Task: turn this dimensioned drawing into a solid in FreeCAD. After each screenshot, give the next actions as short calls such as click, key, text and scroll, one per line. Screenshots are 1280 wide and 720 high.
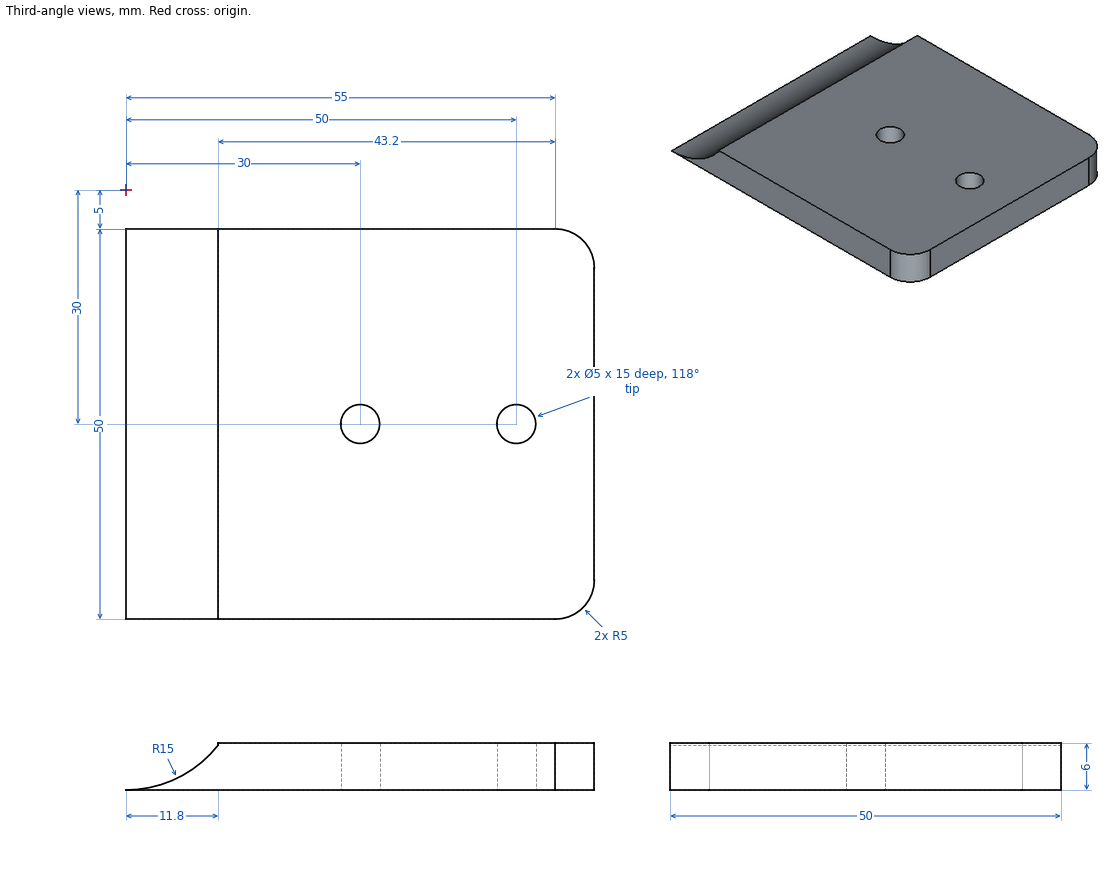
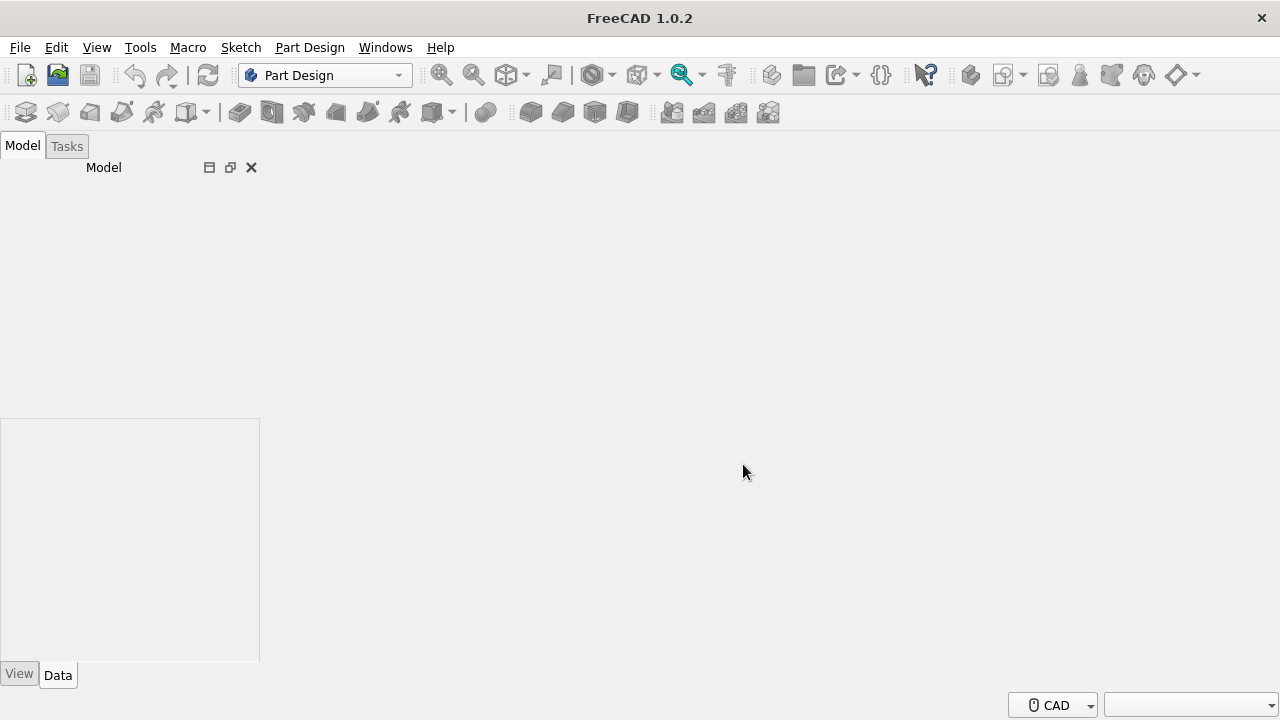
click(26, 76)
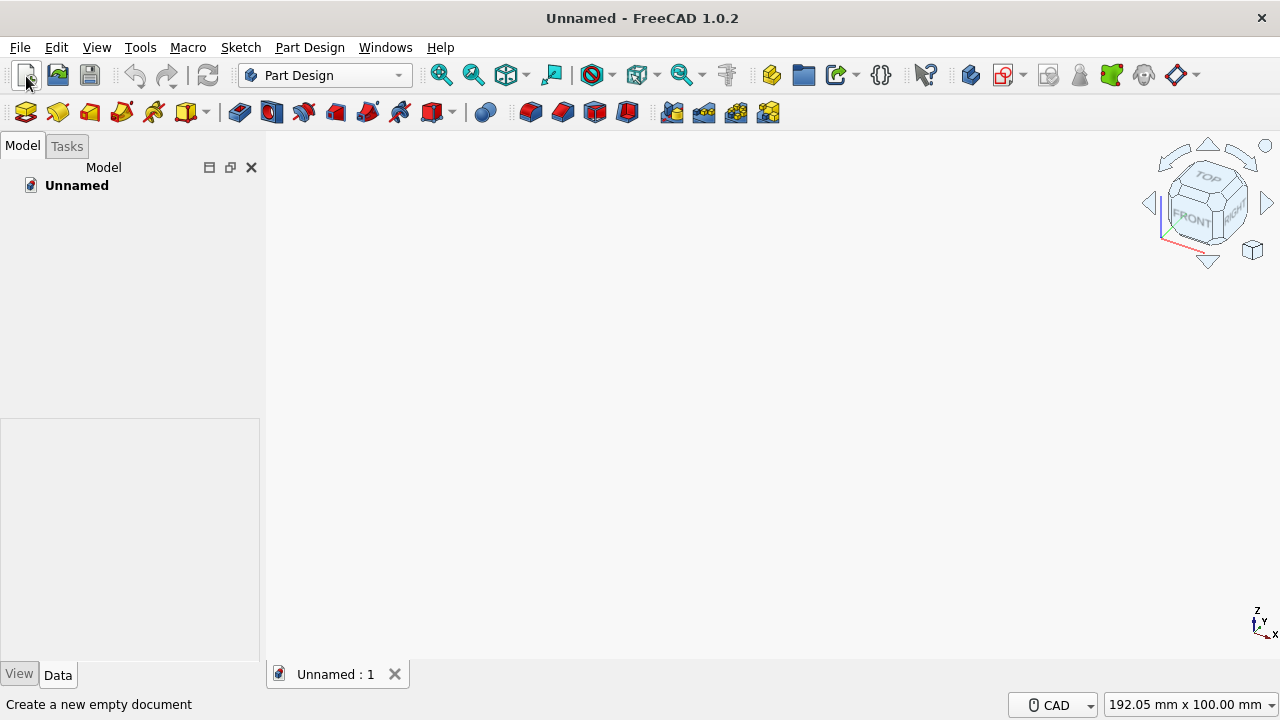
click(972, 76)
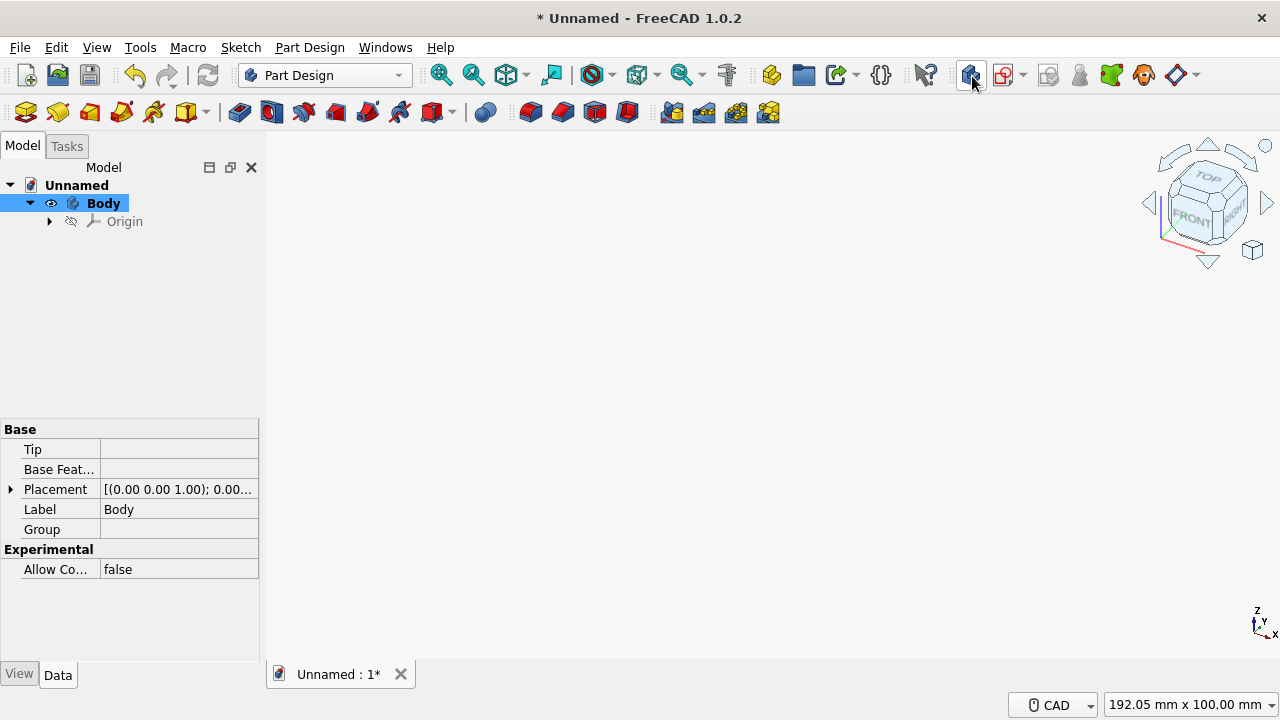
click(50, 221)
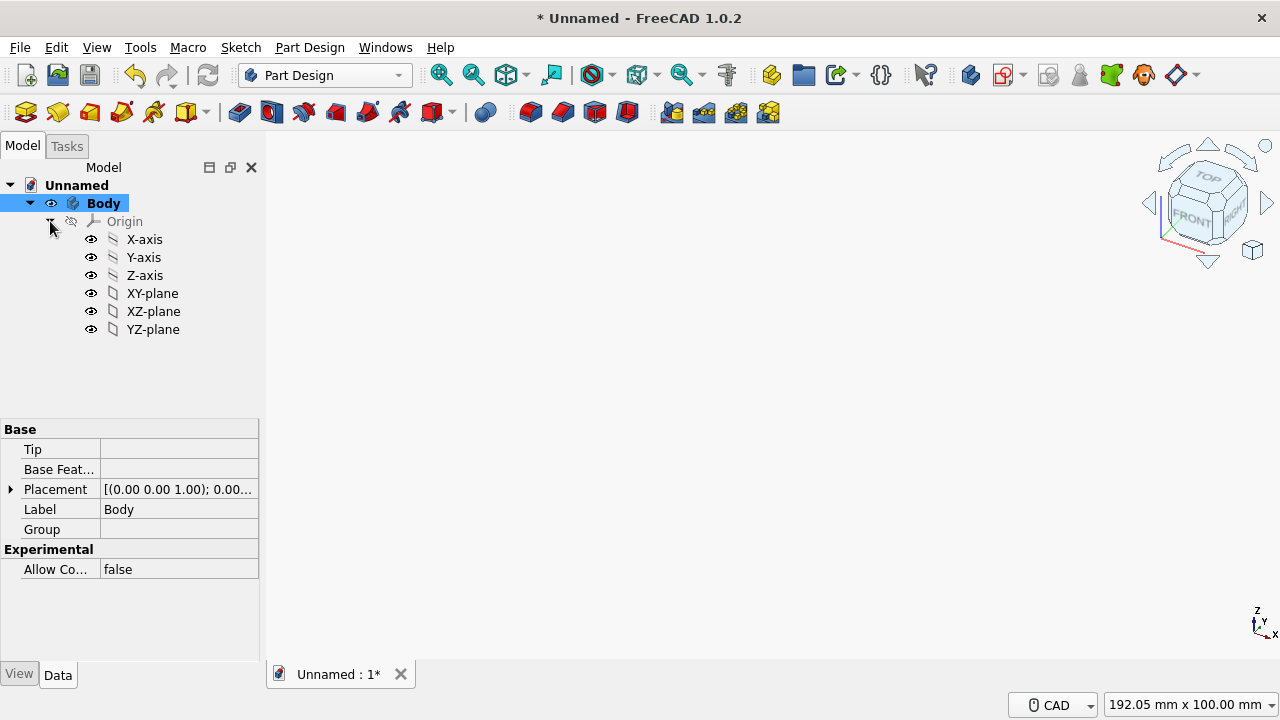
click(136, 293)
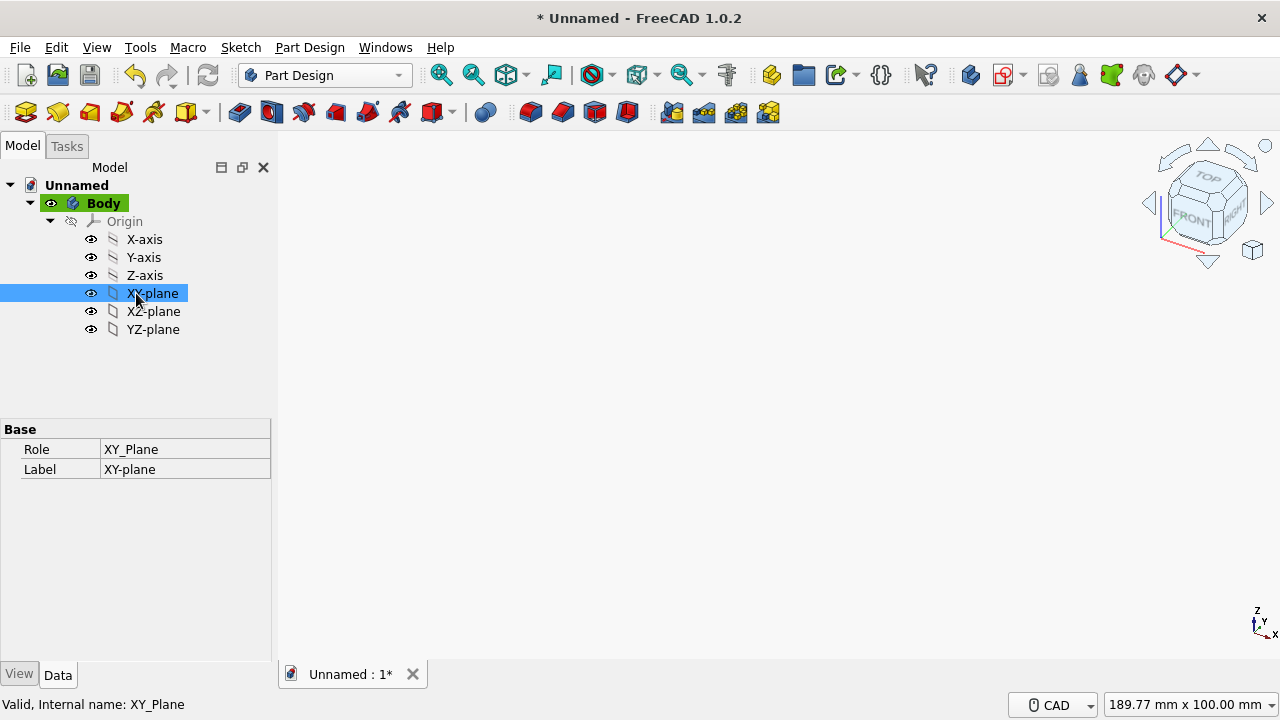
click(1176, 76)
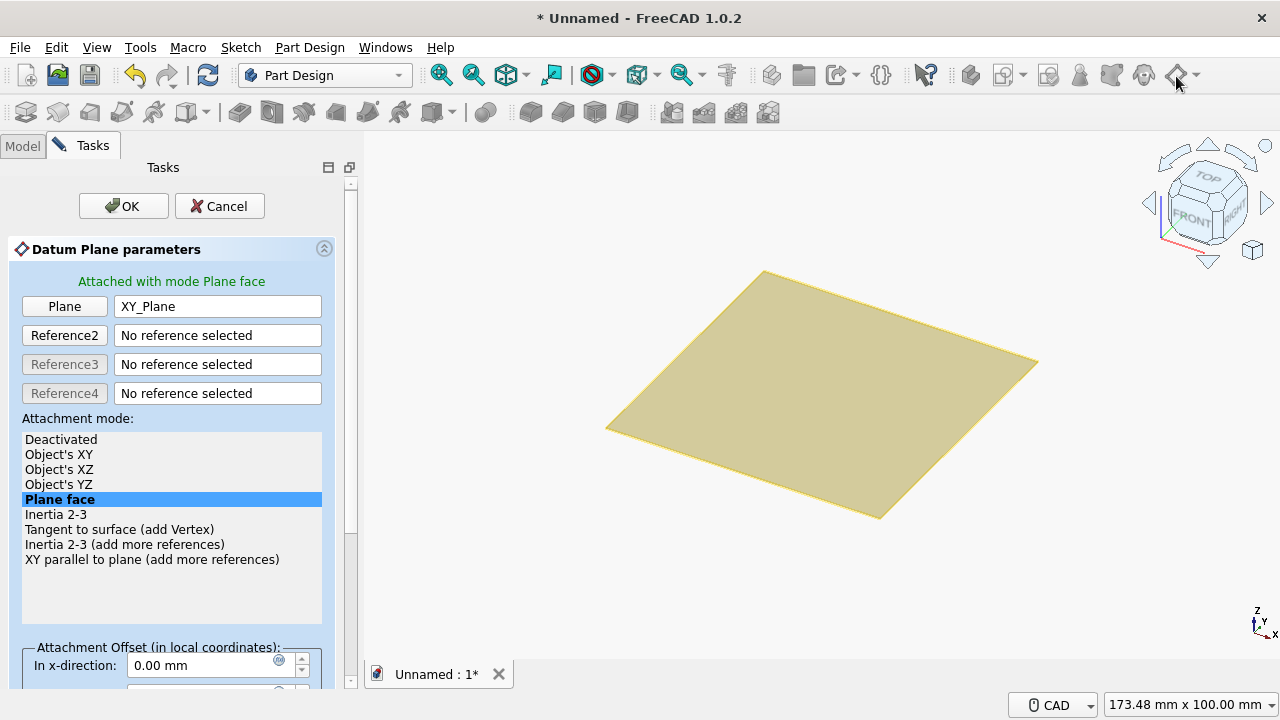
scroll(351, 432, down, 2)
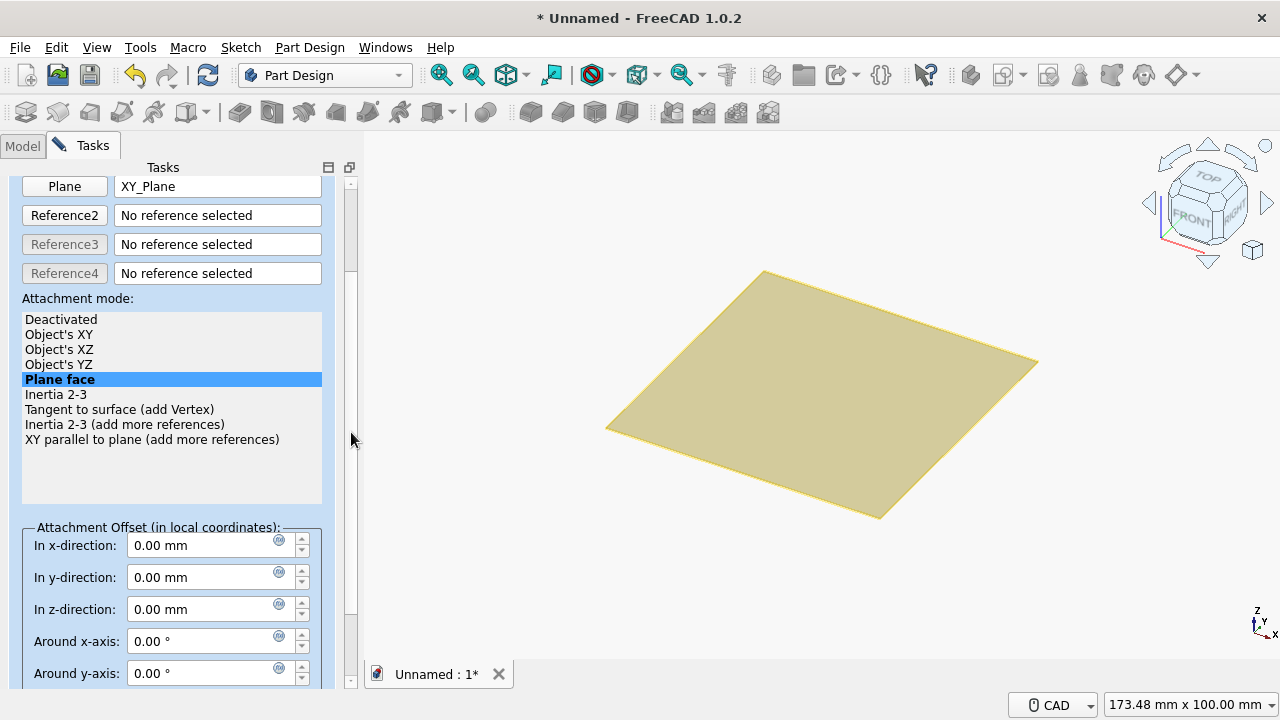
triple_click(210, 609)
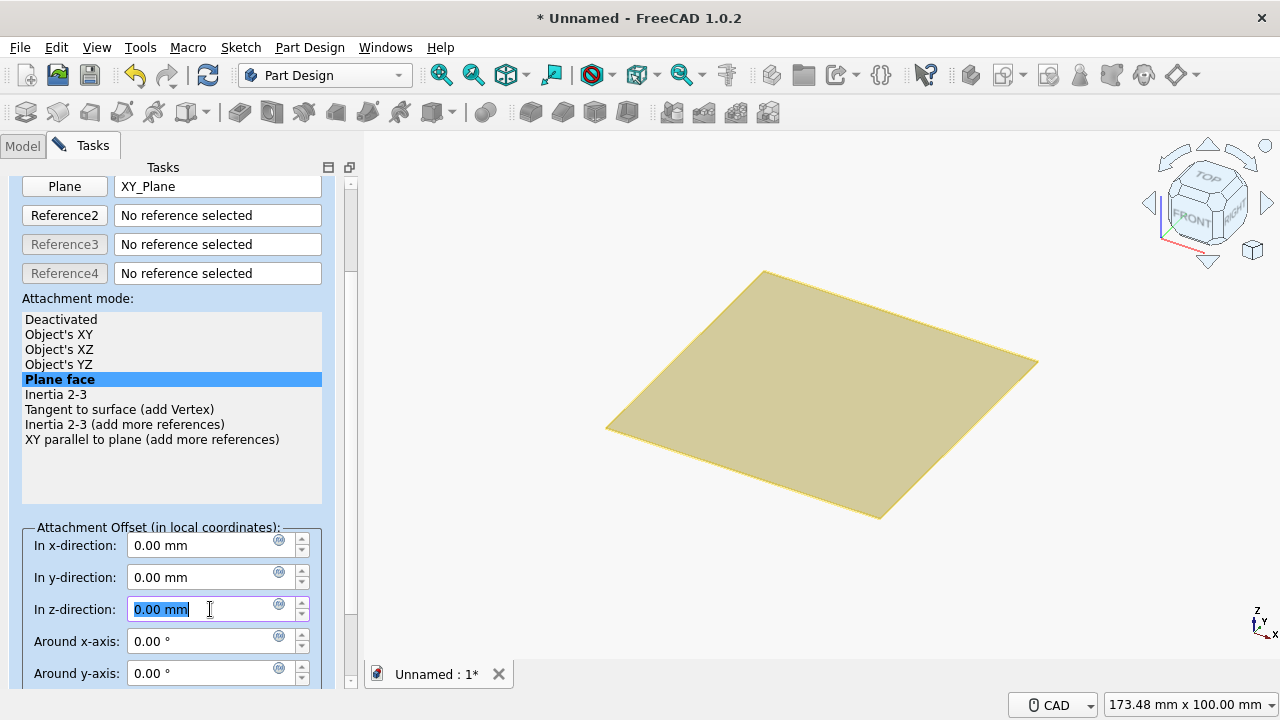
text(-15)
key(Tab)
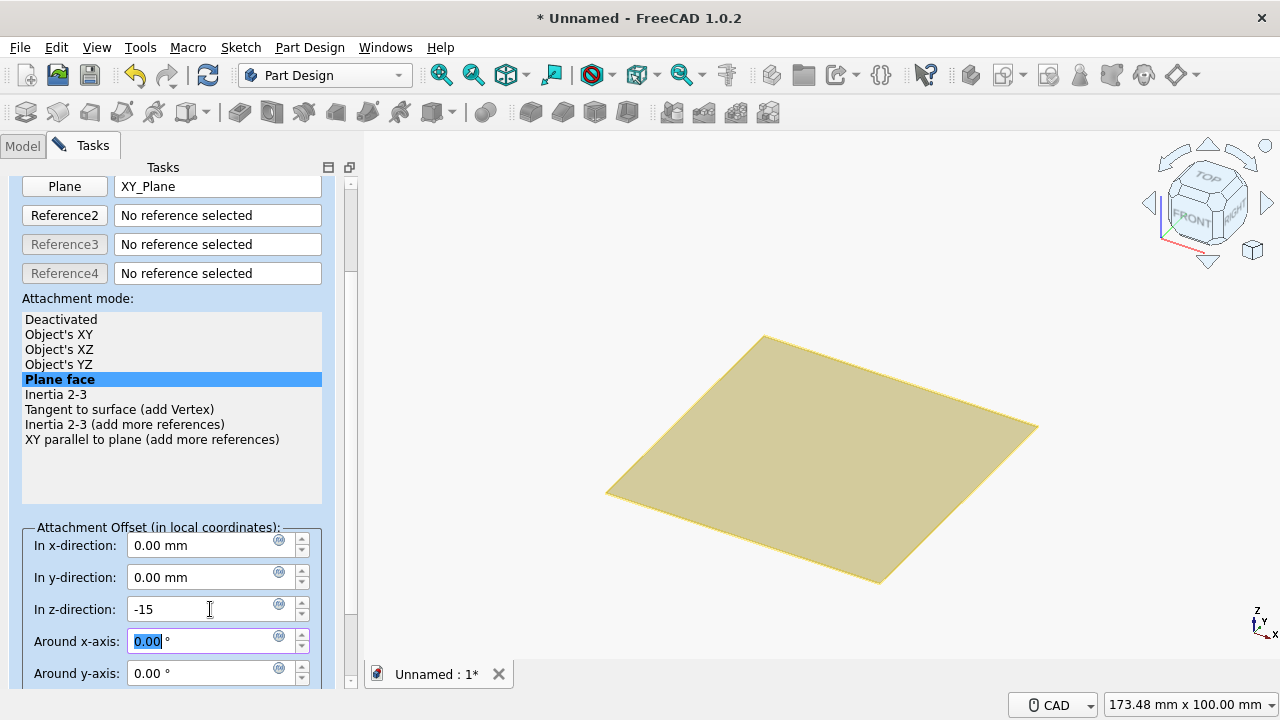
scroll(351, 432, up, 3)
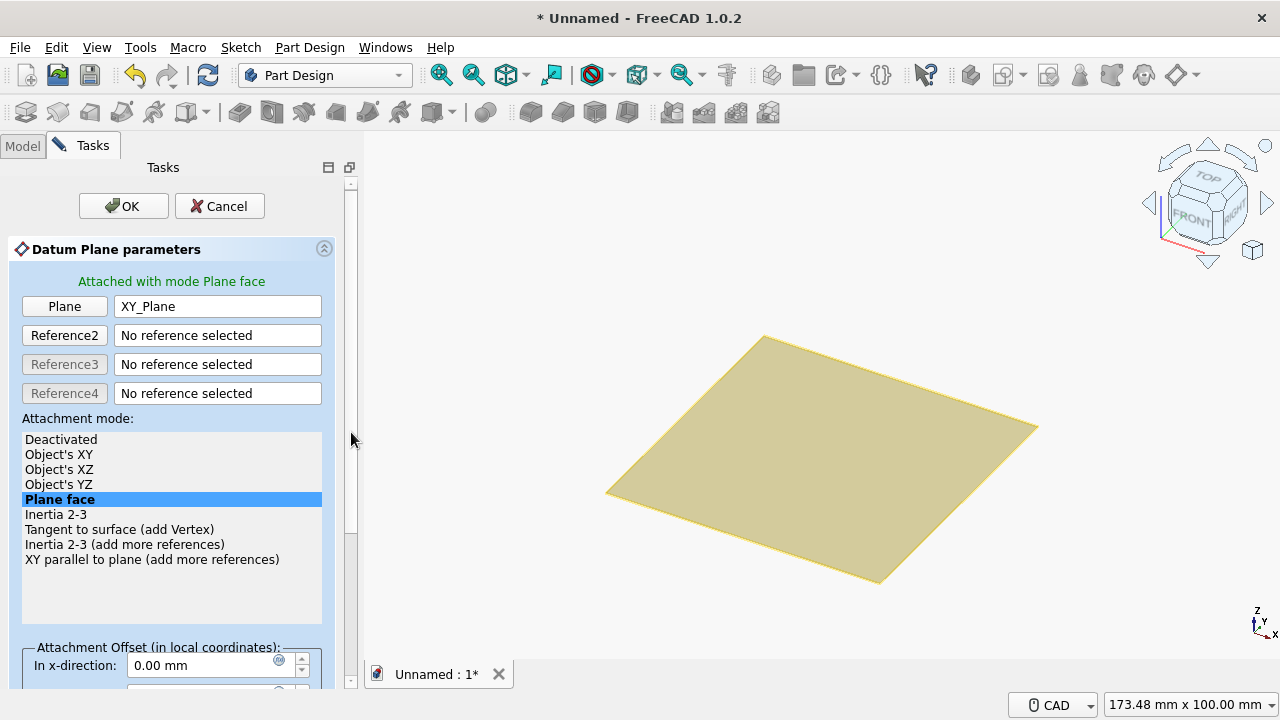
click(124, 206)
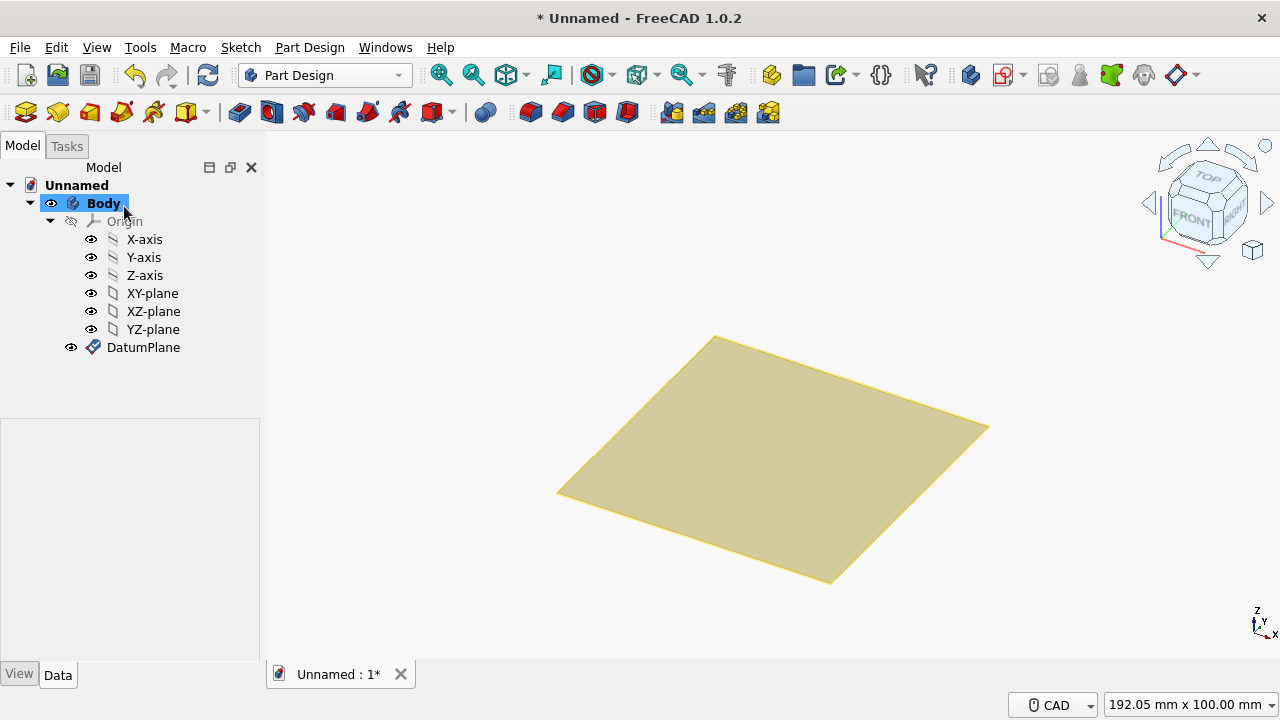
click(116, 347)